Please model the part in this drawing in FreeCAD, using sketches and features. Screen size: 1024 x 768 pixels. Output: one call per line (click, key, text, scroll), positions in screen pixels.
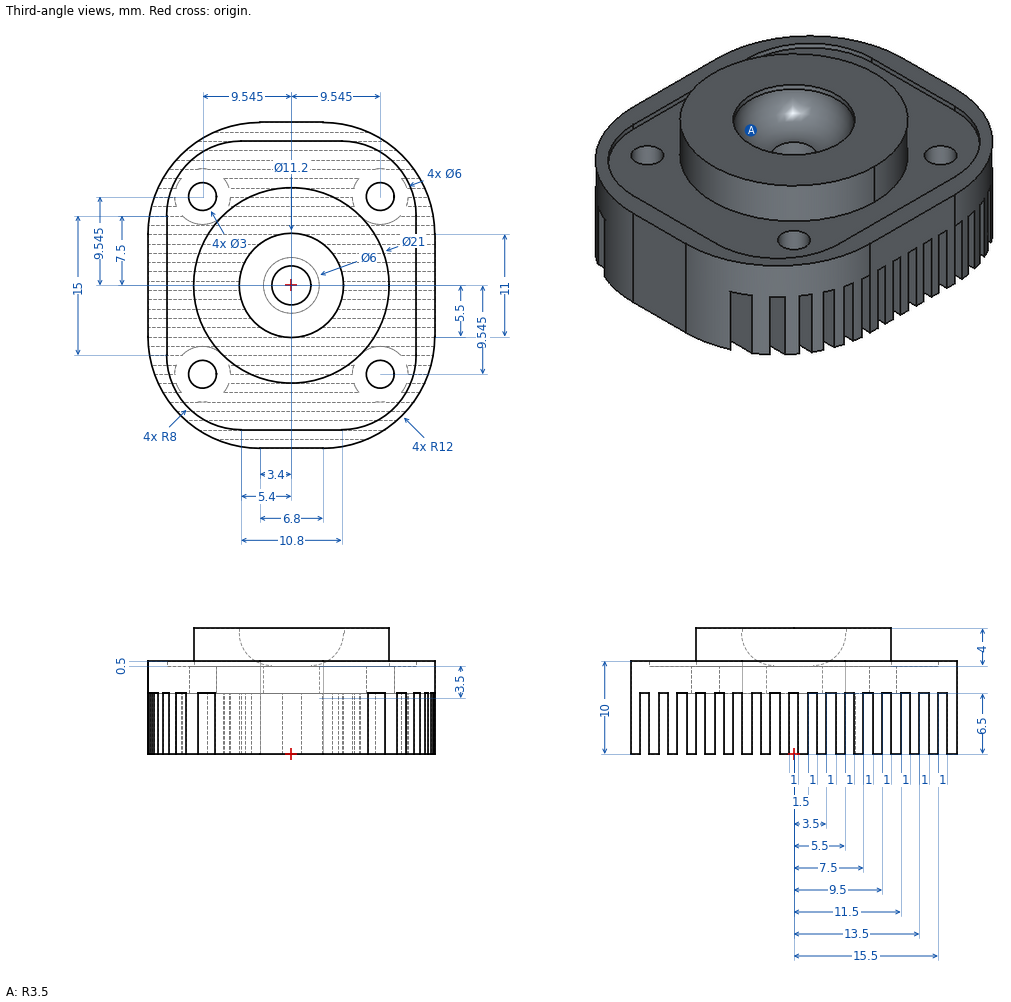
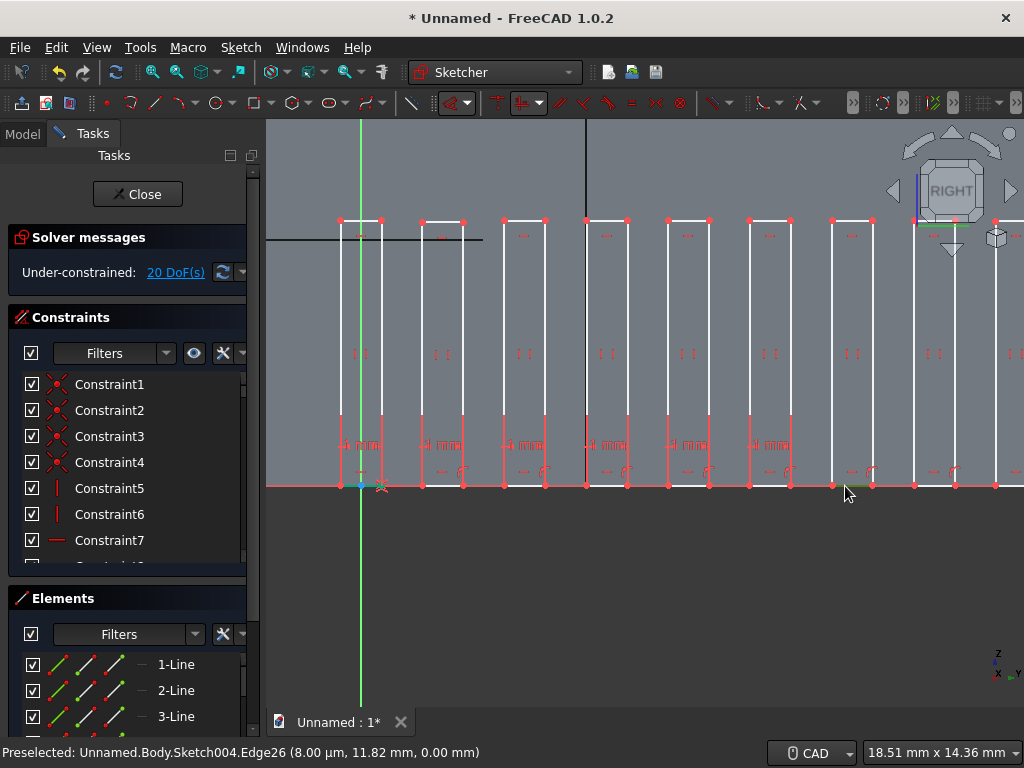
key(l)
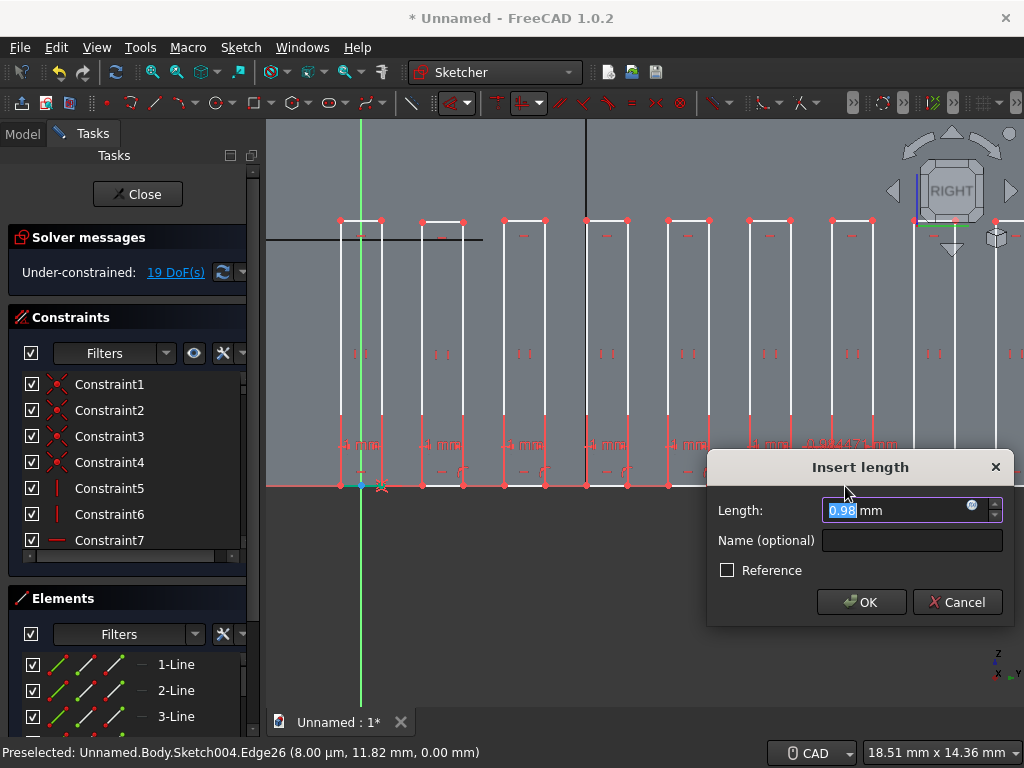
text(1)
key(Return)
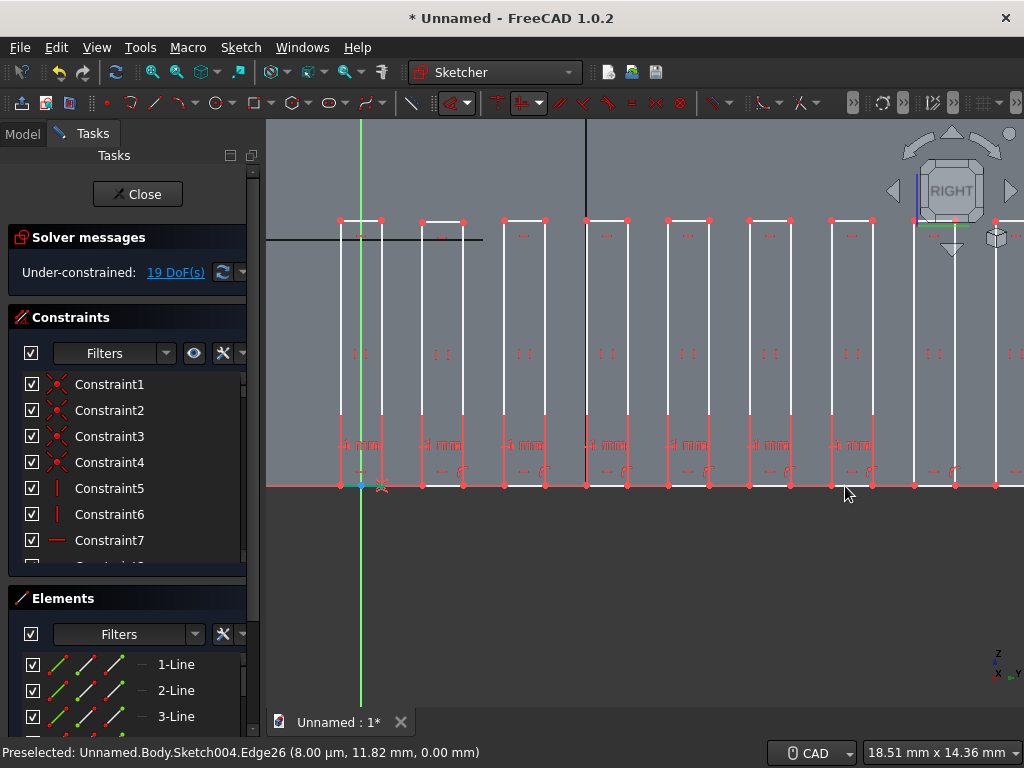
scroll(440, 486, down, 3)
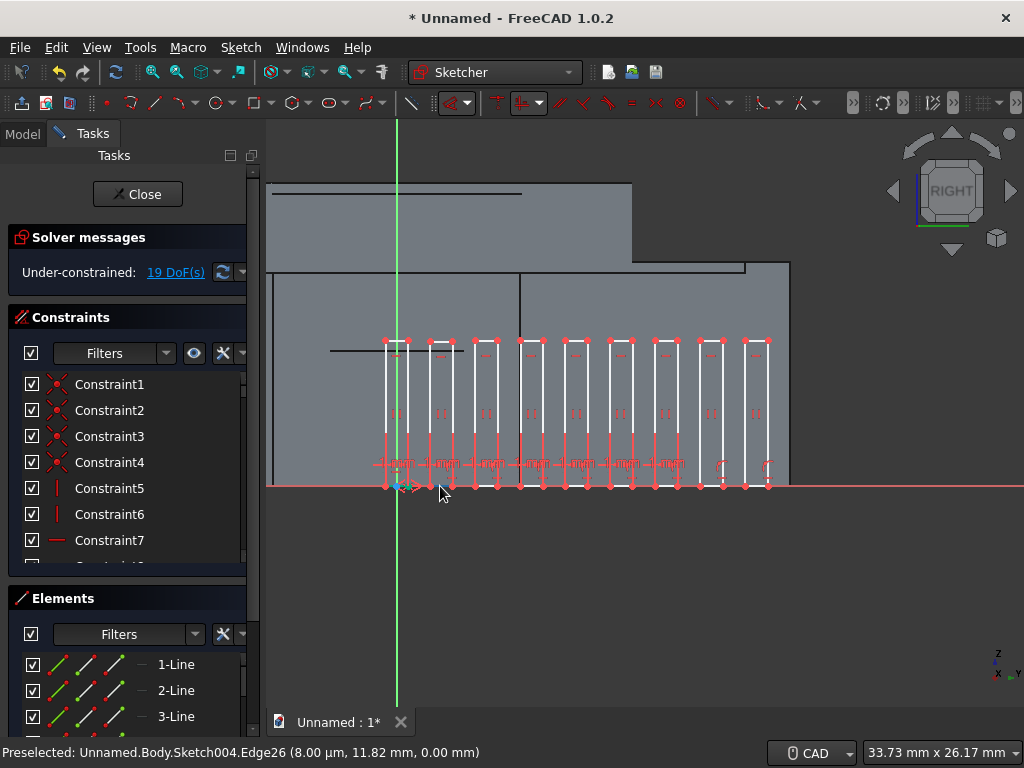
scroll(707, 486, up, 4)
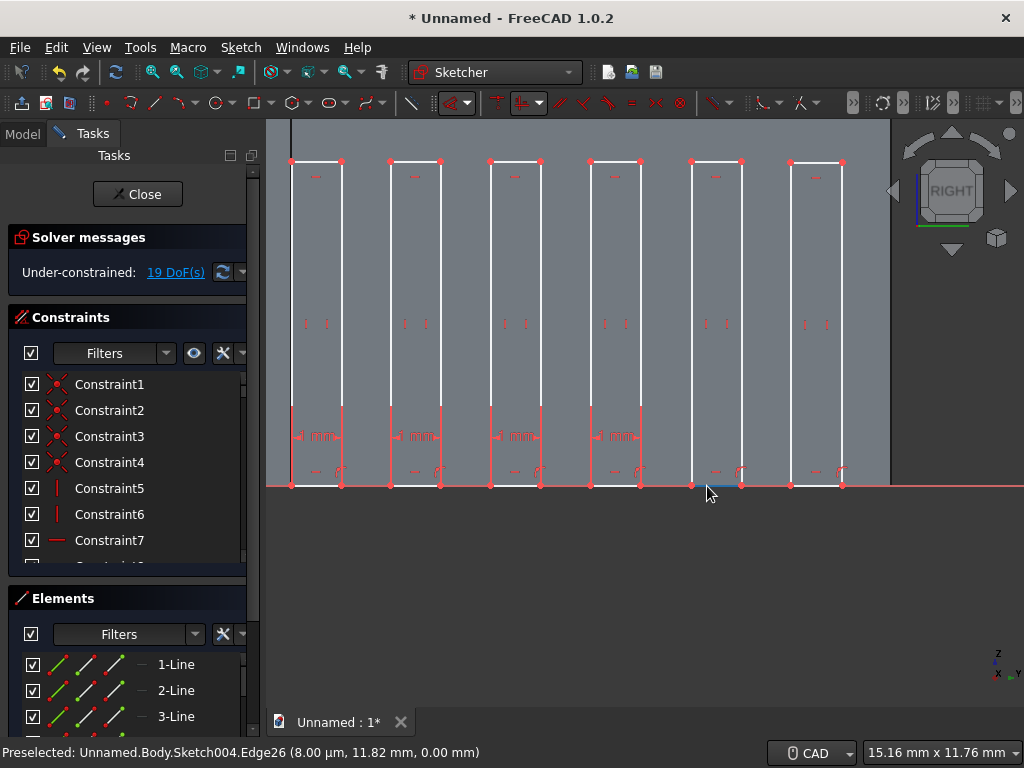
click(707, 486)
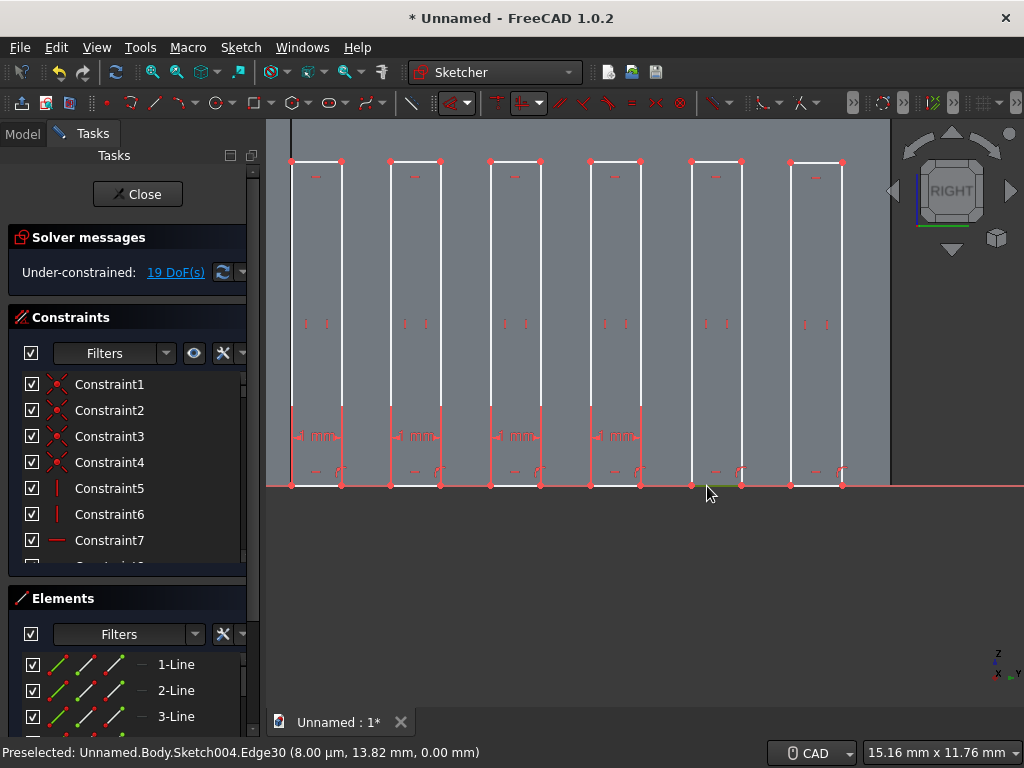
click(470, 104)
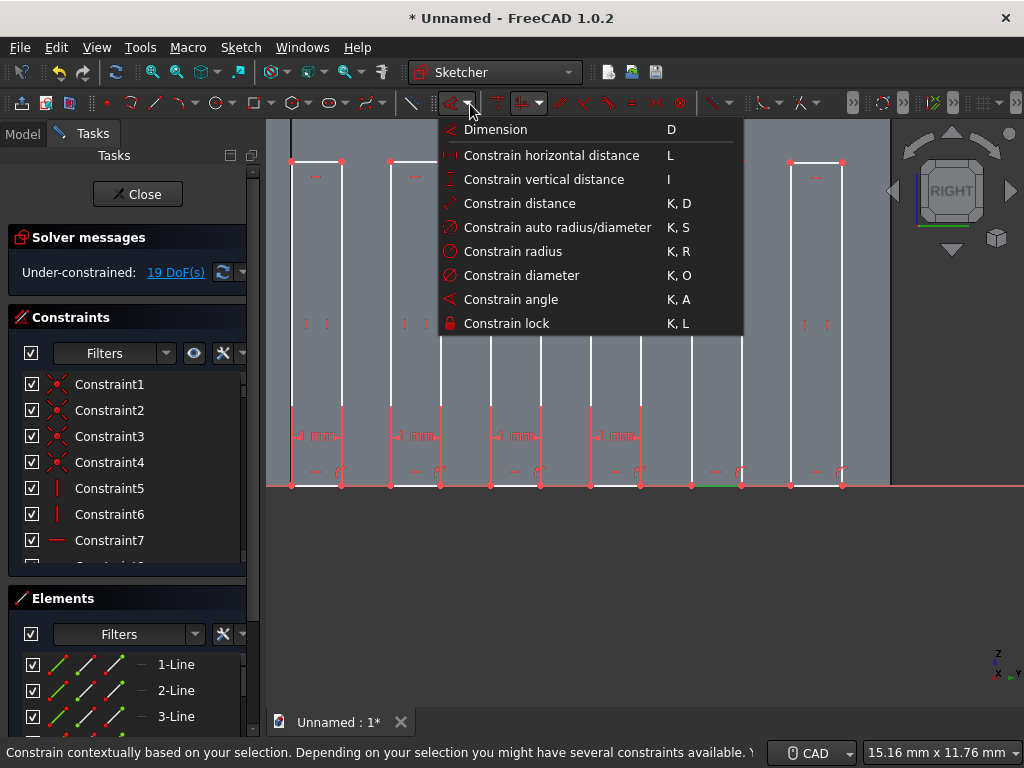
click(591, 155)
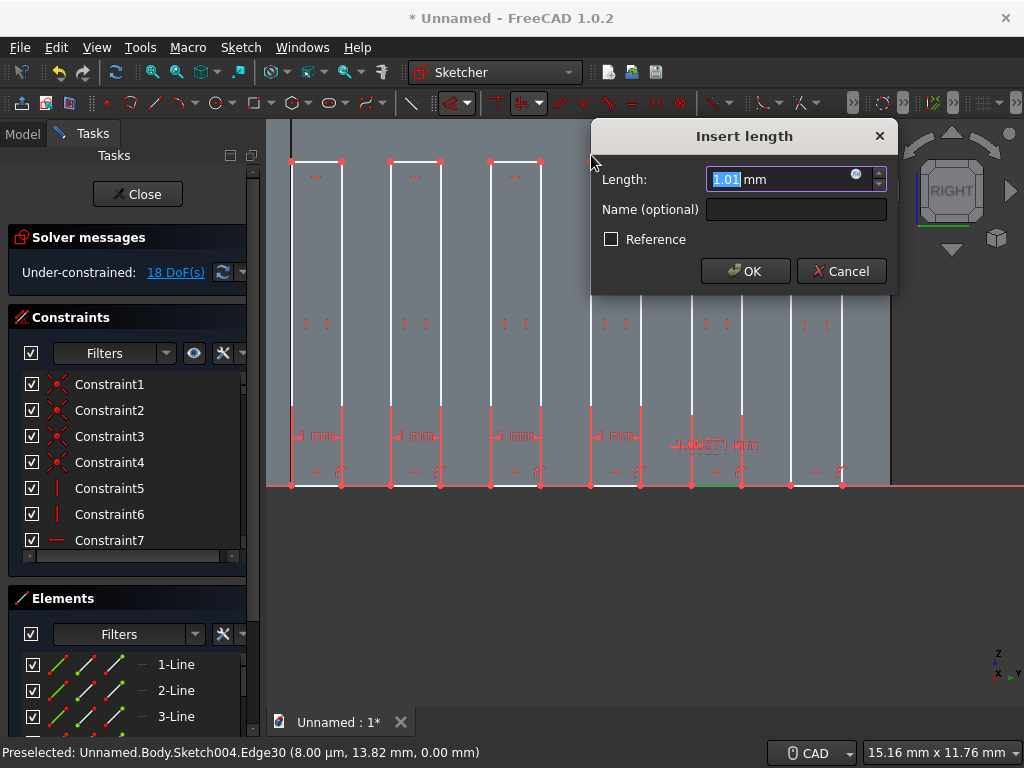
text(1)
key(Return)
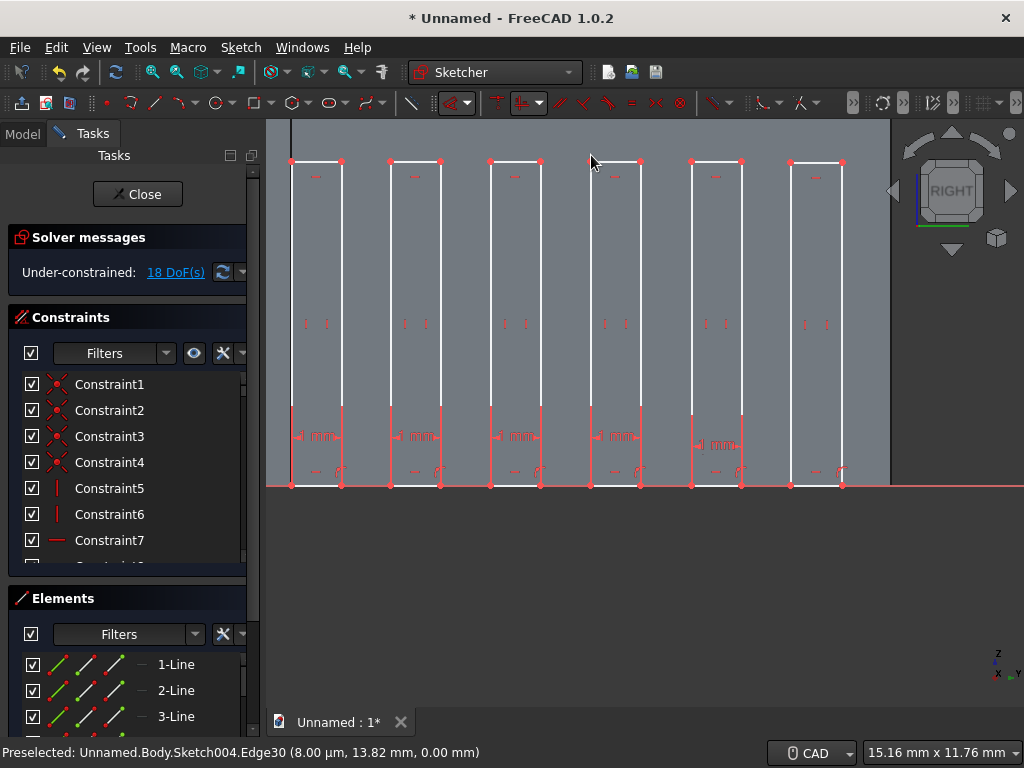
click(806, 486)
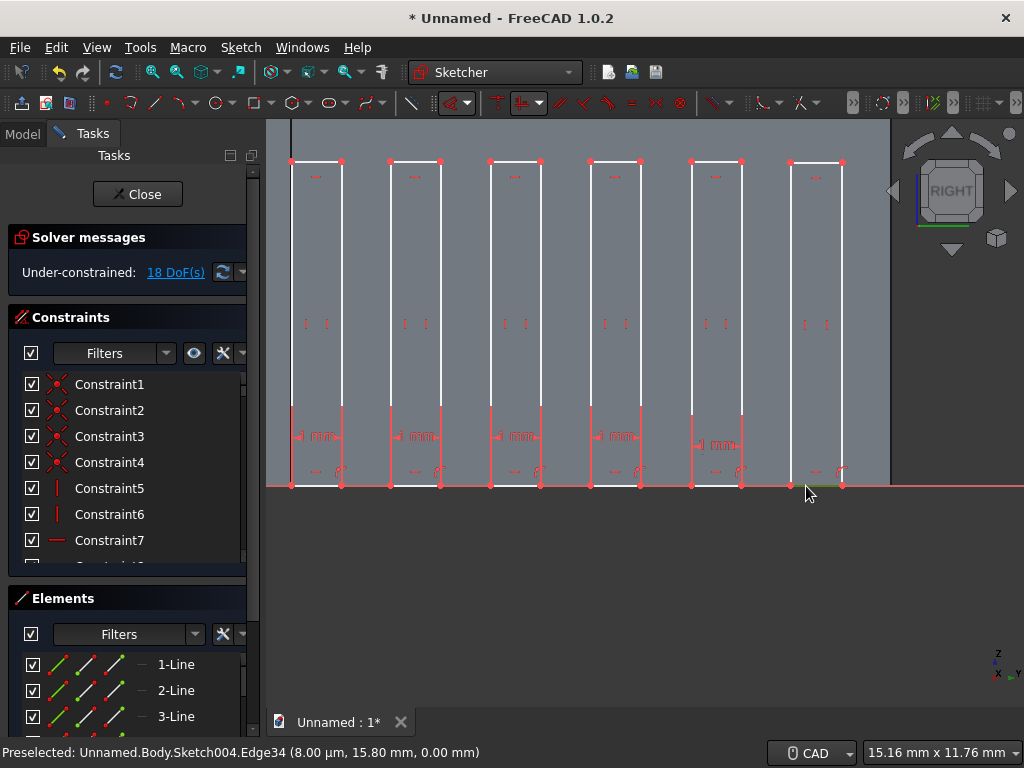
key(l)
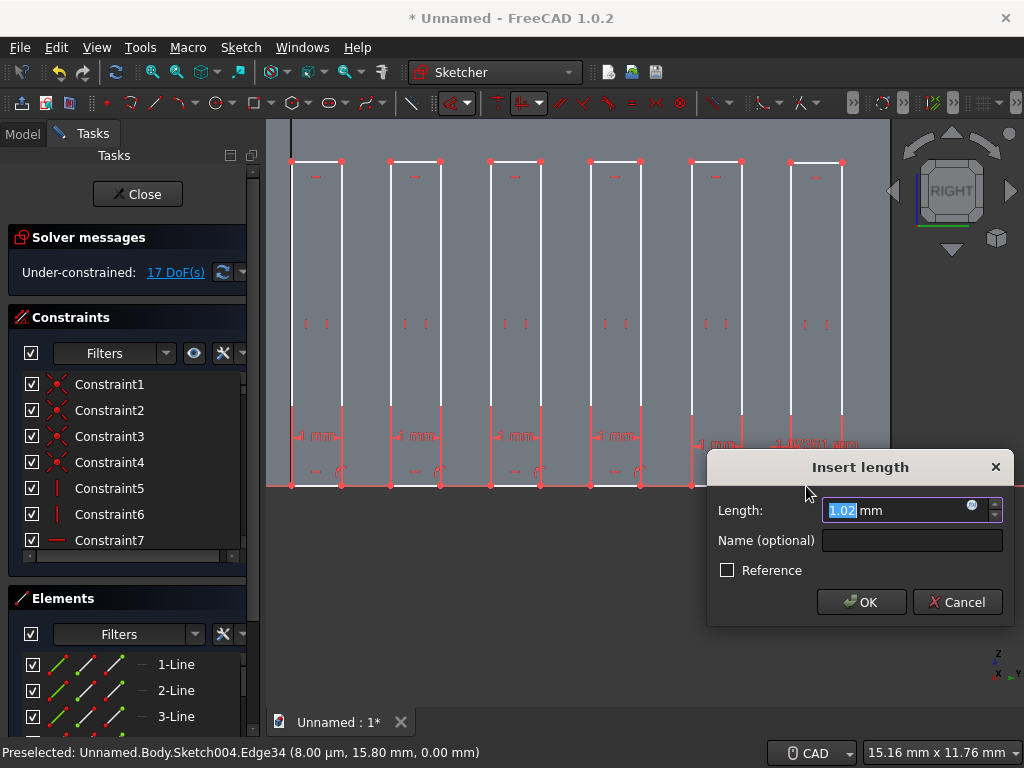
text(1)
key(Return)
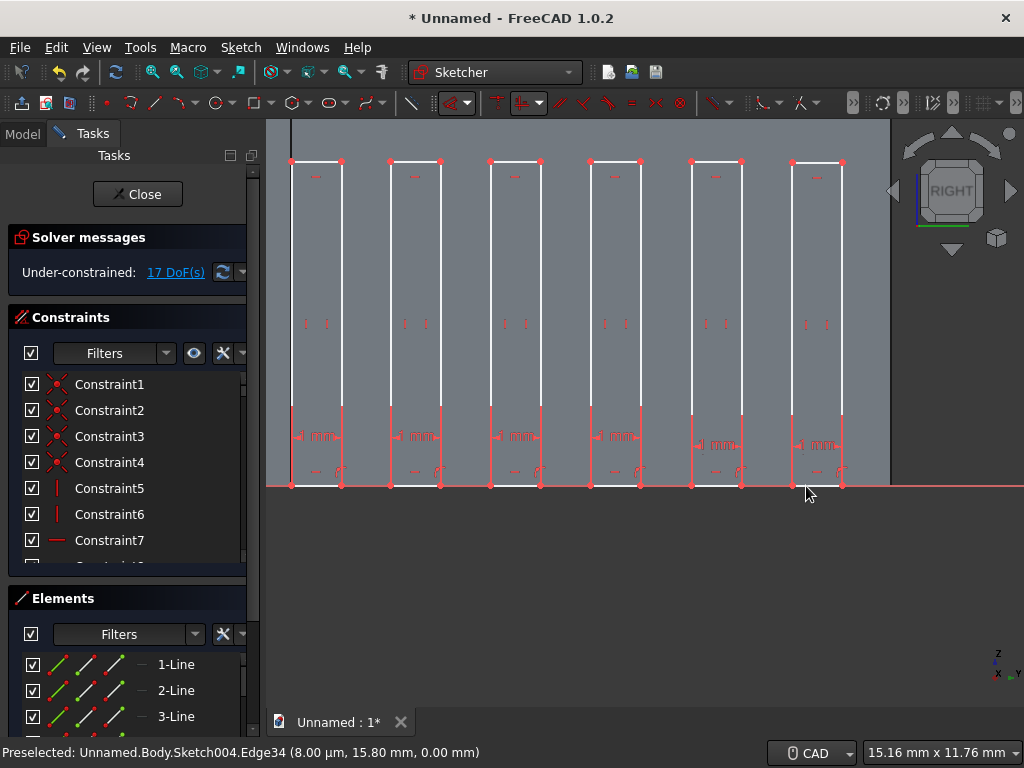
scroll(707, 486, down, 4)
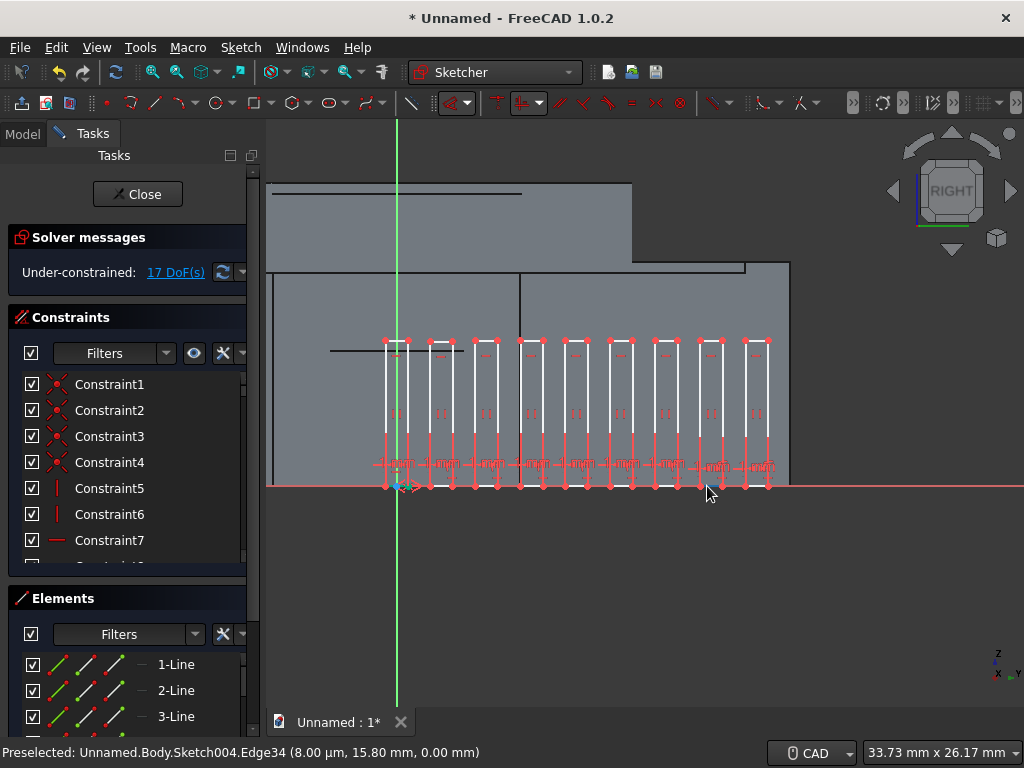
click(430, 385)